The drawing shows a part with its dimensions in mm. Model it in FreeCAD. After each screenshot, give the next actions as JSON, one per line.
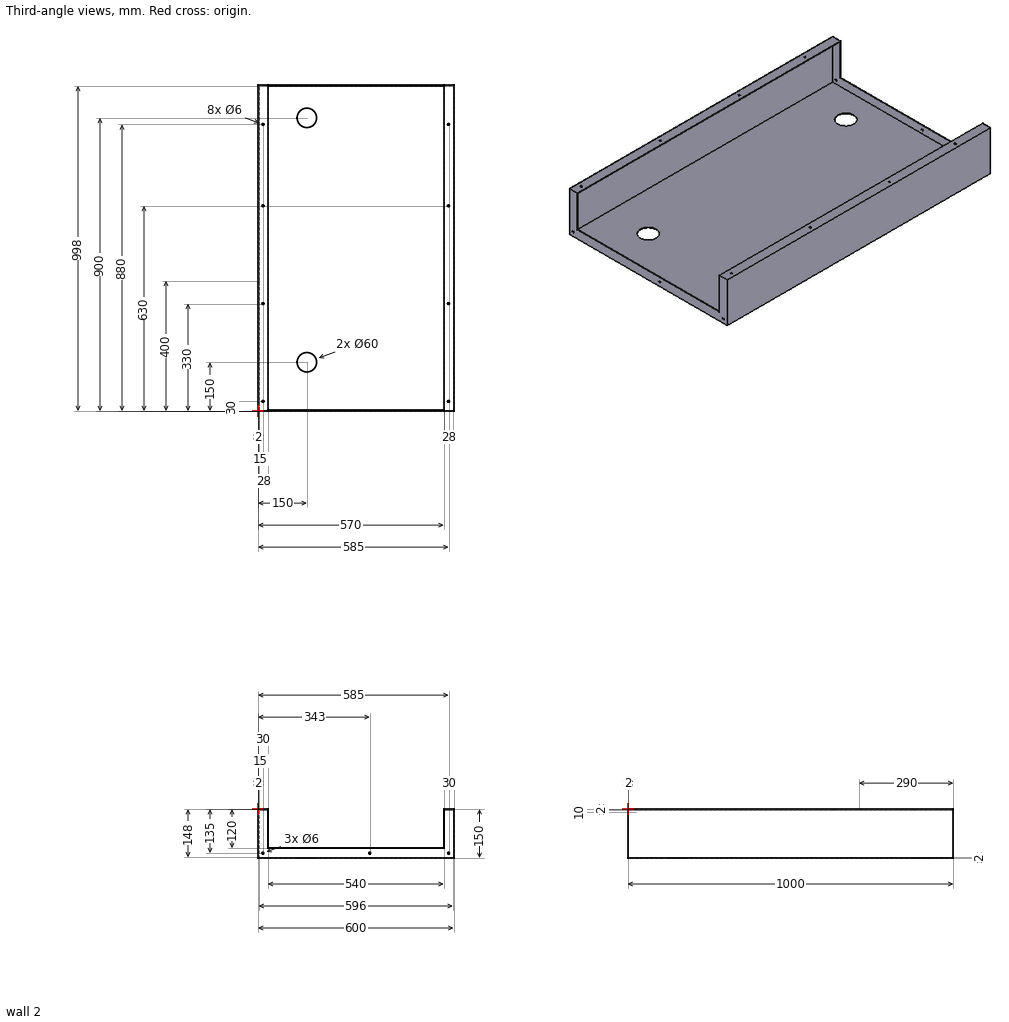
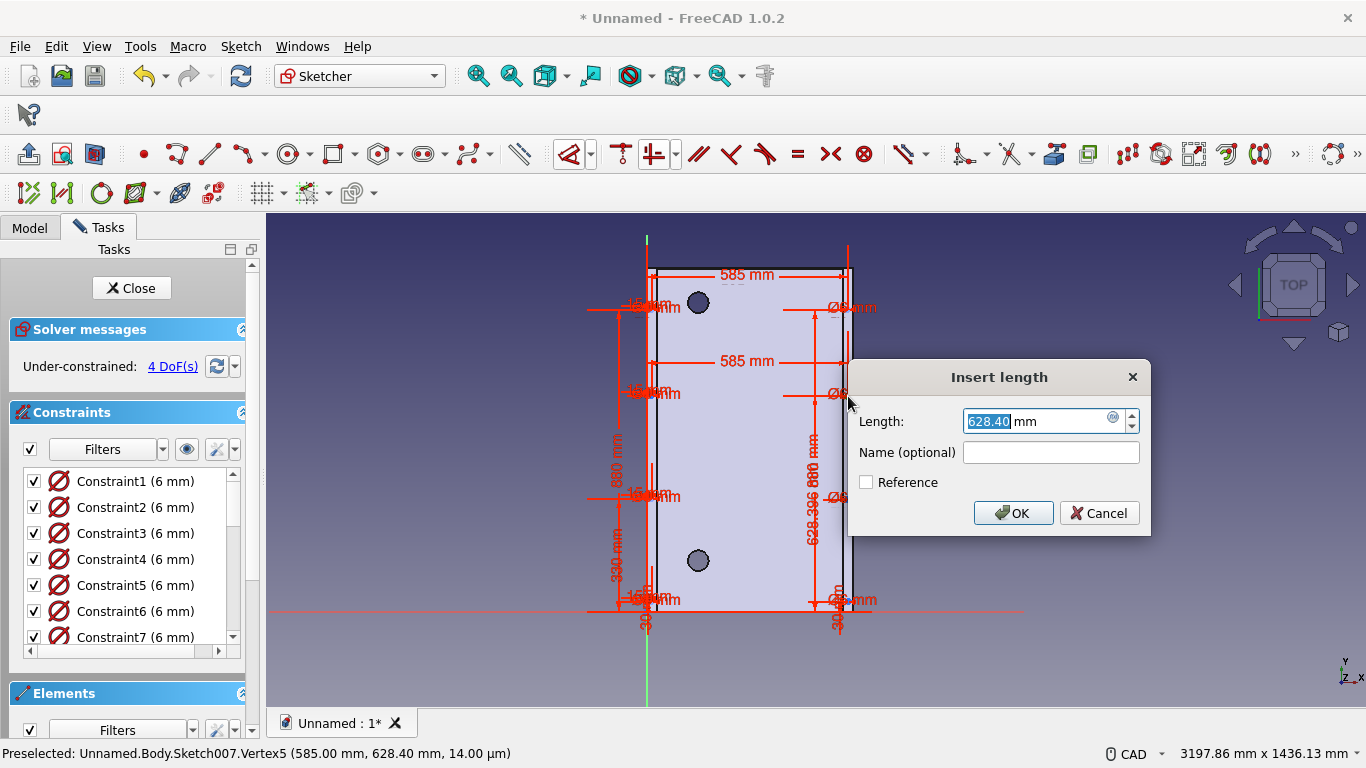
{"action": "type", "text": "630"}
{"action": "key", "text": "Return"}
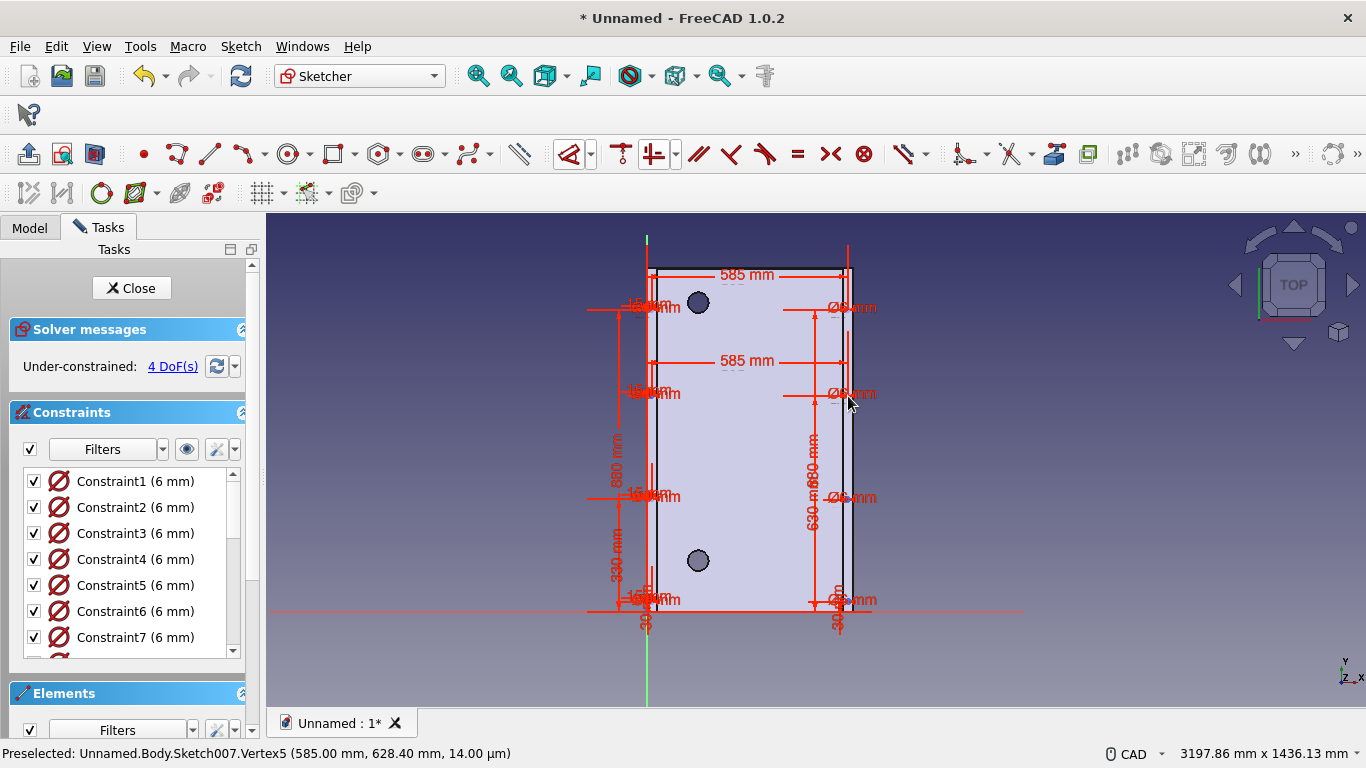
{"action": "left_click", "coordinate": [652, 396]}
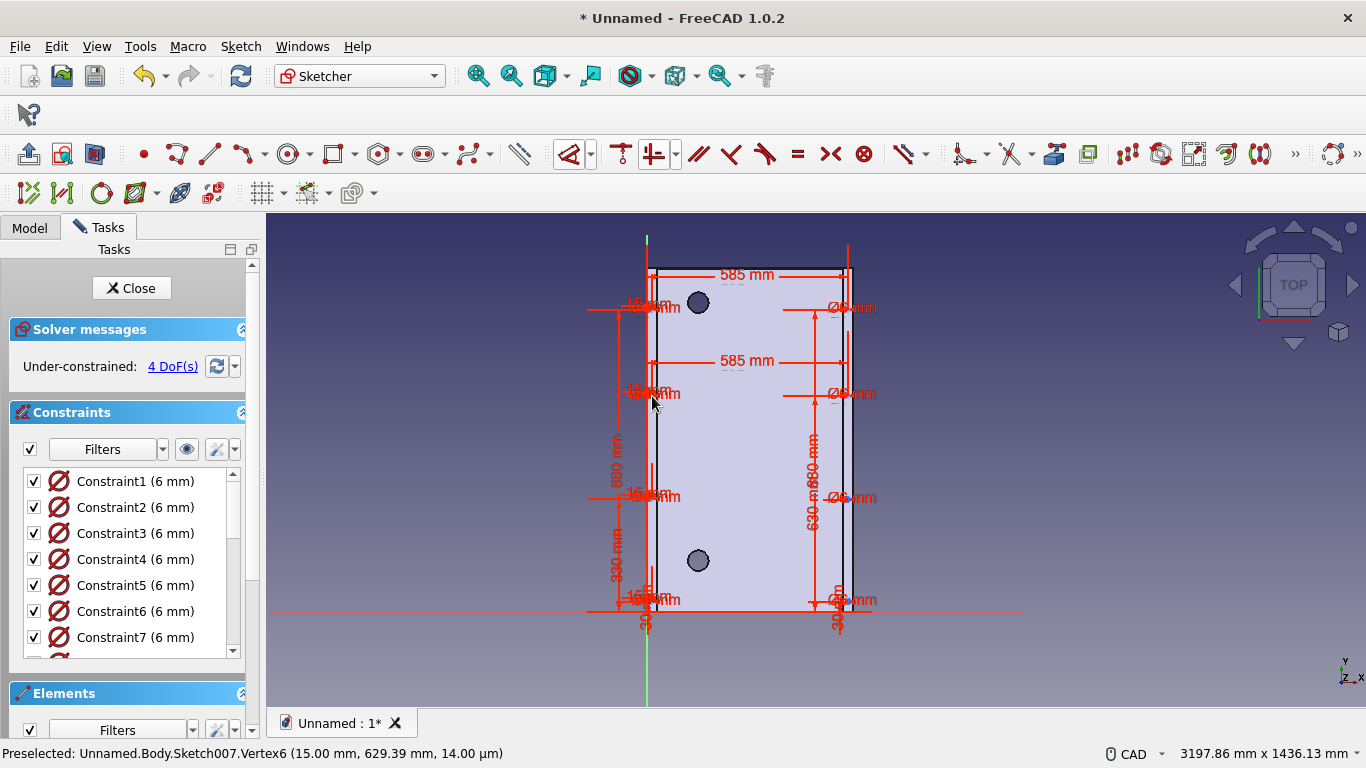
{"action": "key", "text": "i"}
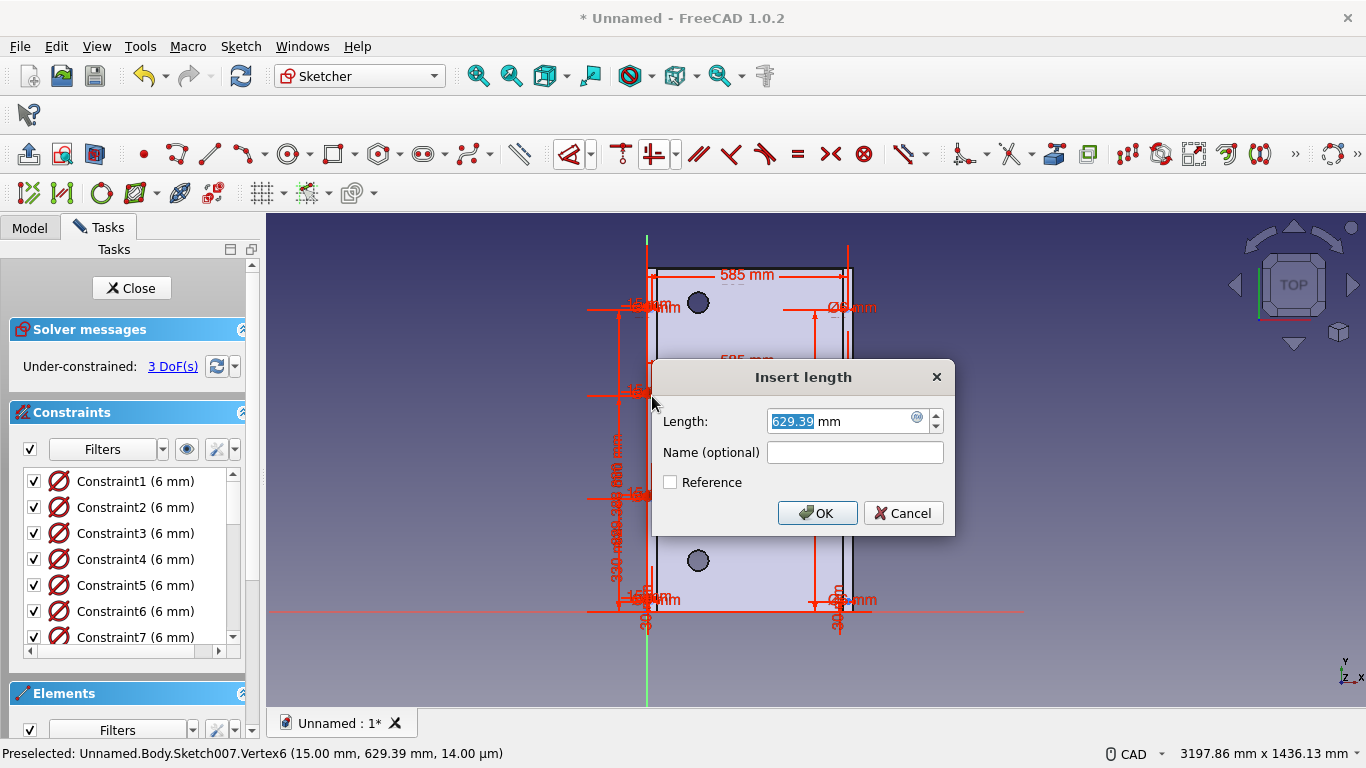
{"action": "type", "text": "630"}
{"action": "key", "text": "Return"}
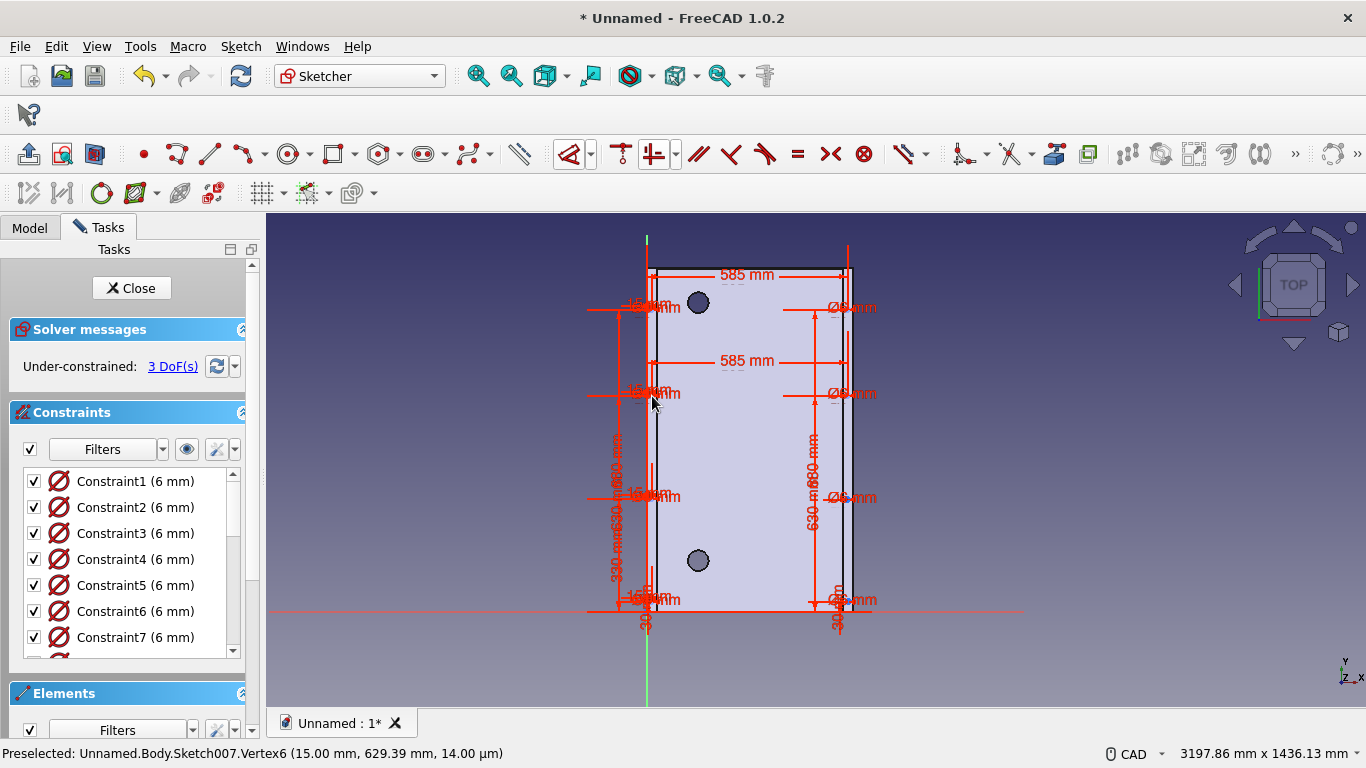
{"action": "left_click", "coordinate": [848, 500]}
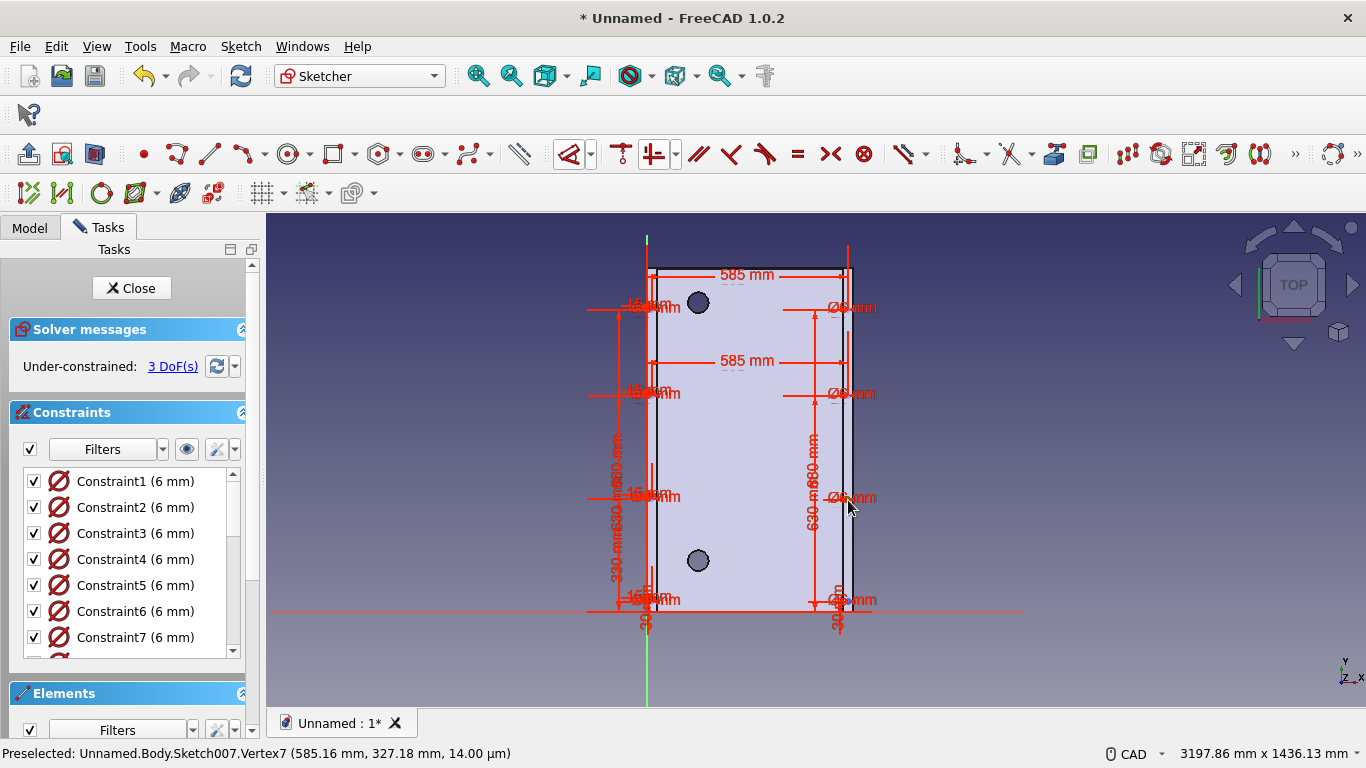
{"action": "left_click", "coordinate": [590, 154]}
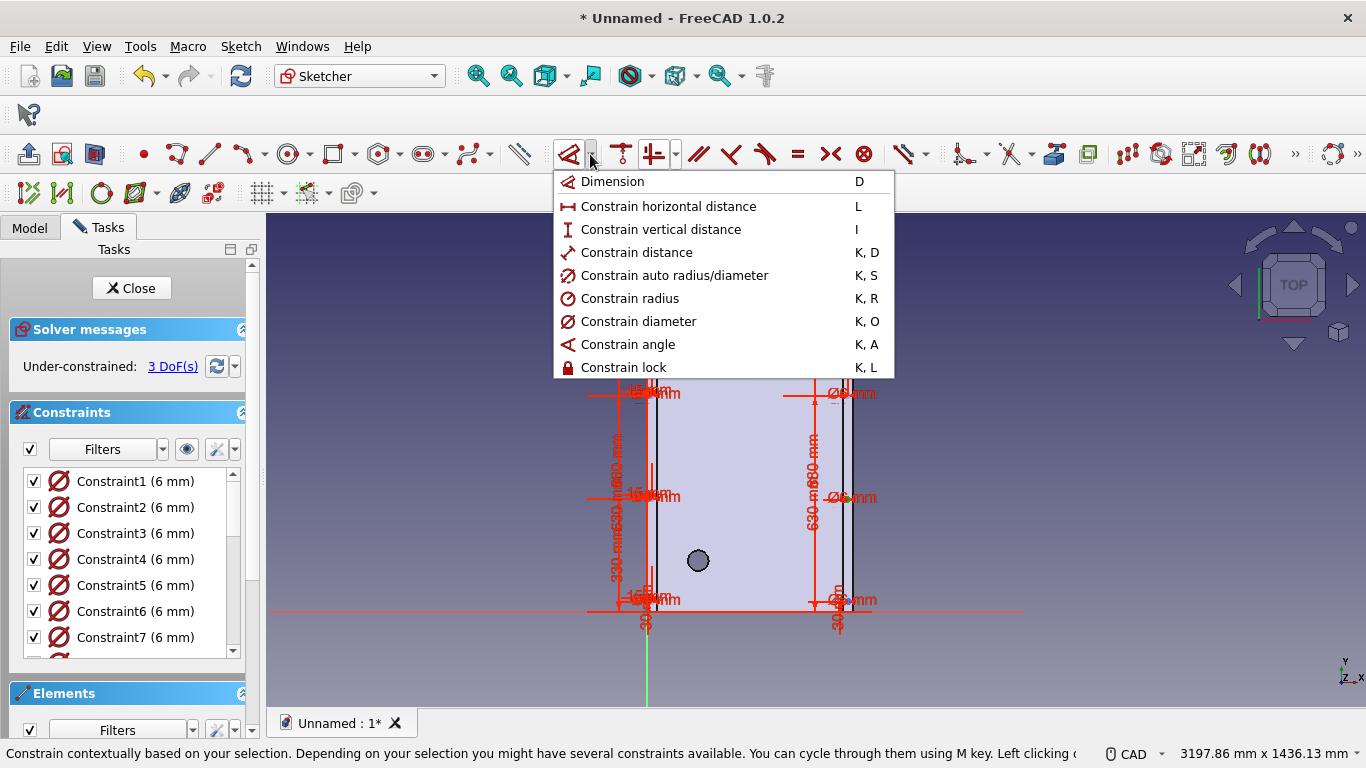
{"action": "left_click", "coordinate": [724, 206]}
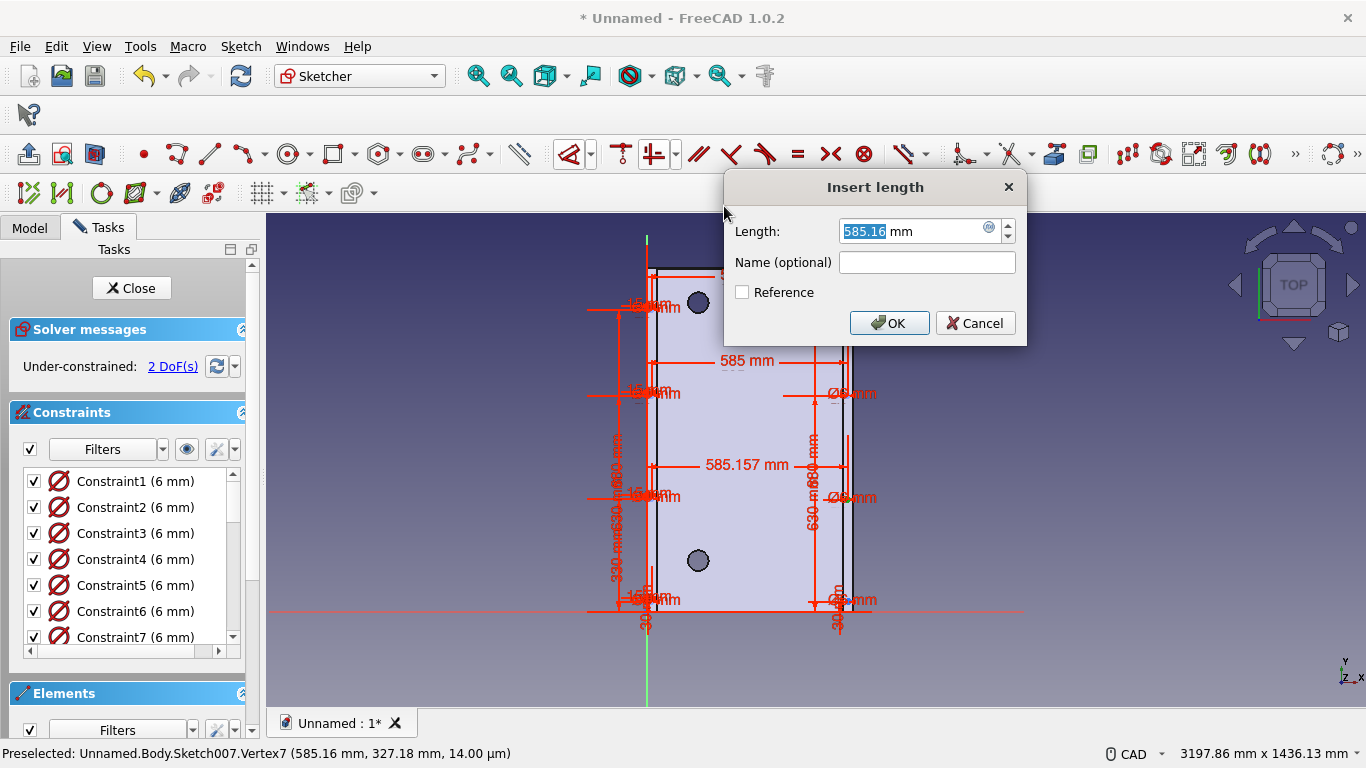
{"action": "type", "text": "585"}
{"action": "key", "text": "Return"}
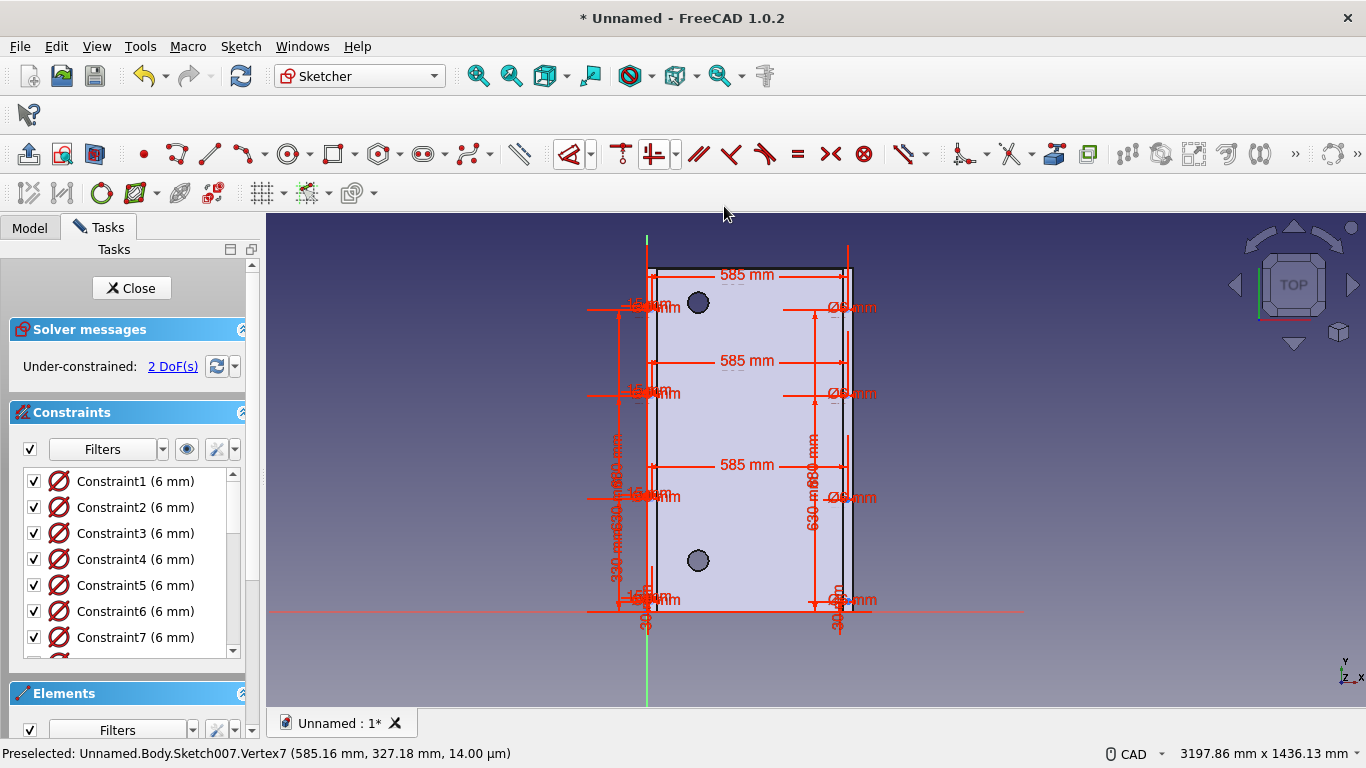
{"action": "left_click", "coordinate": [848, 500]}